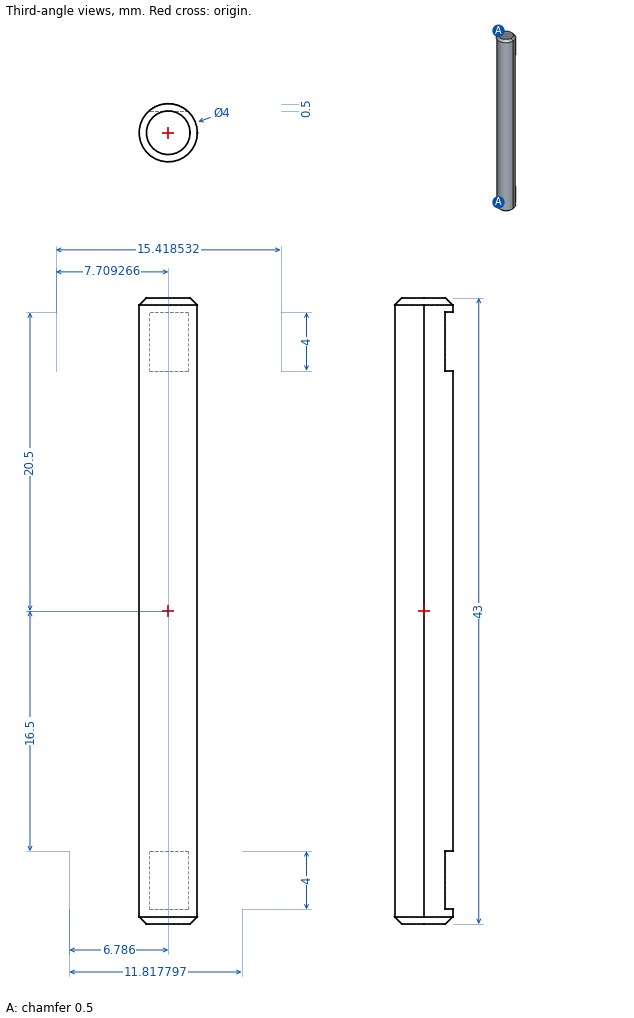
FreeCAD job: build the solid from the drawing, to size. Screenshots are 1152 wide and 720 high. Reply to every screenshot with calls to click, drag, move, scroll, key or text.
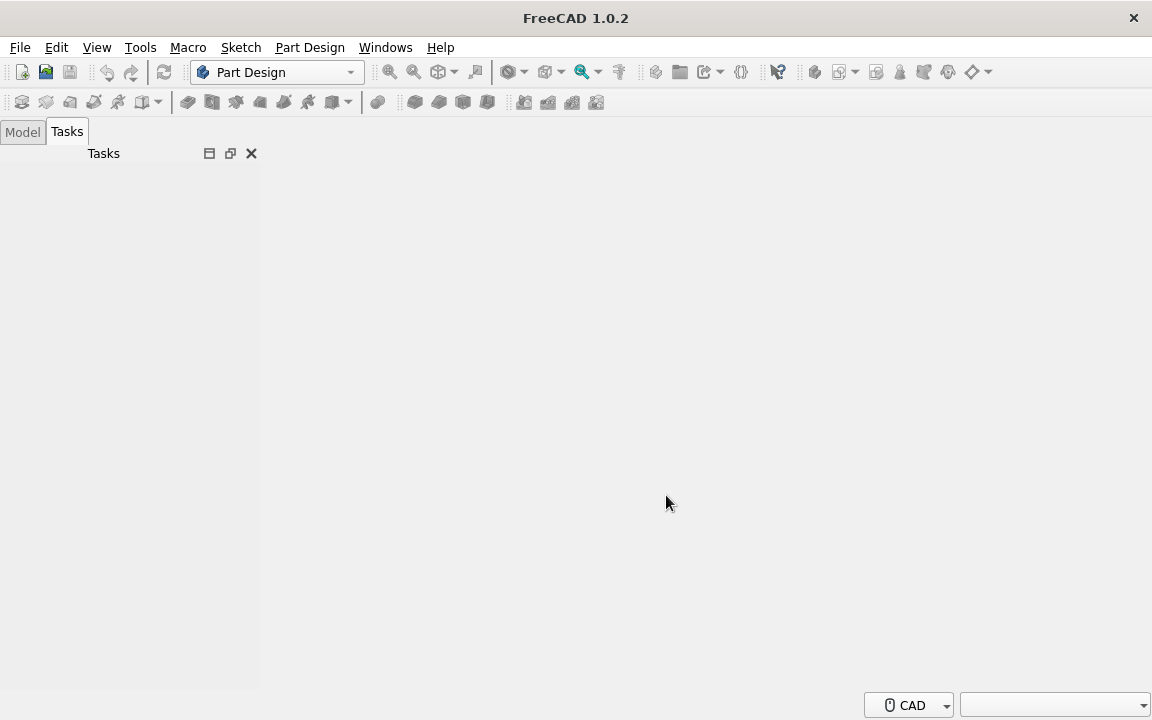
key(ctrl+n)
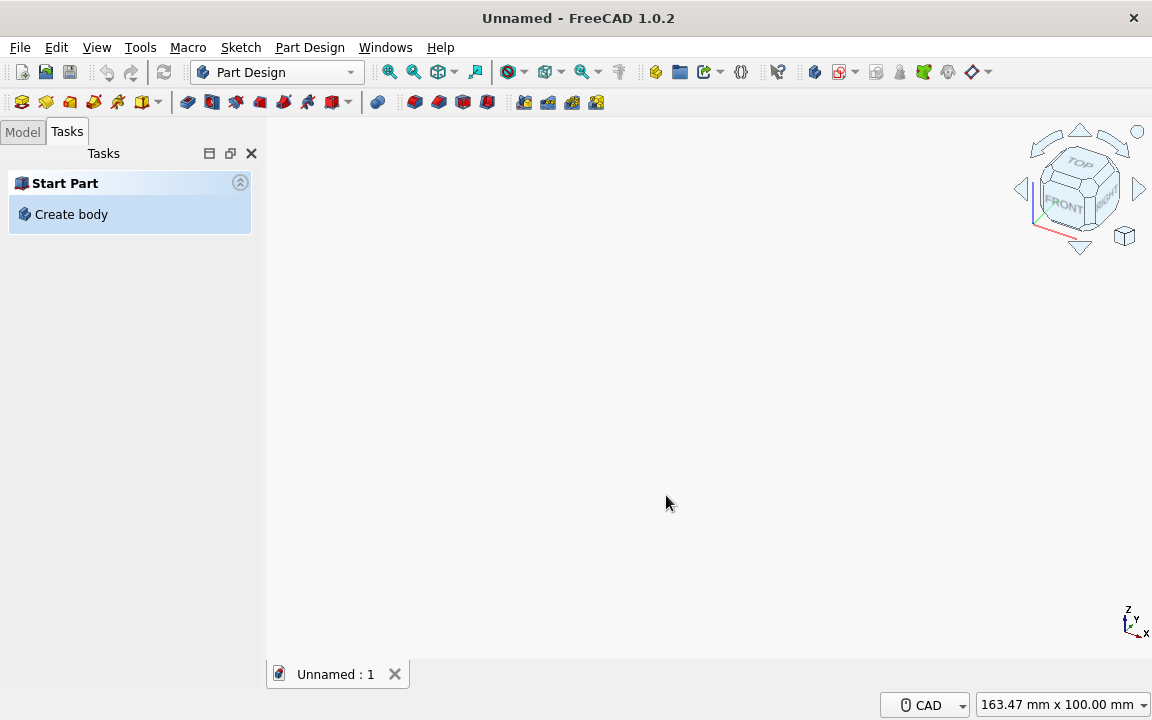
click(840, 72)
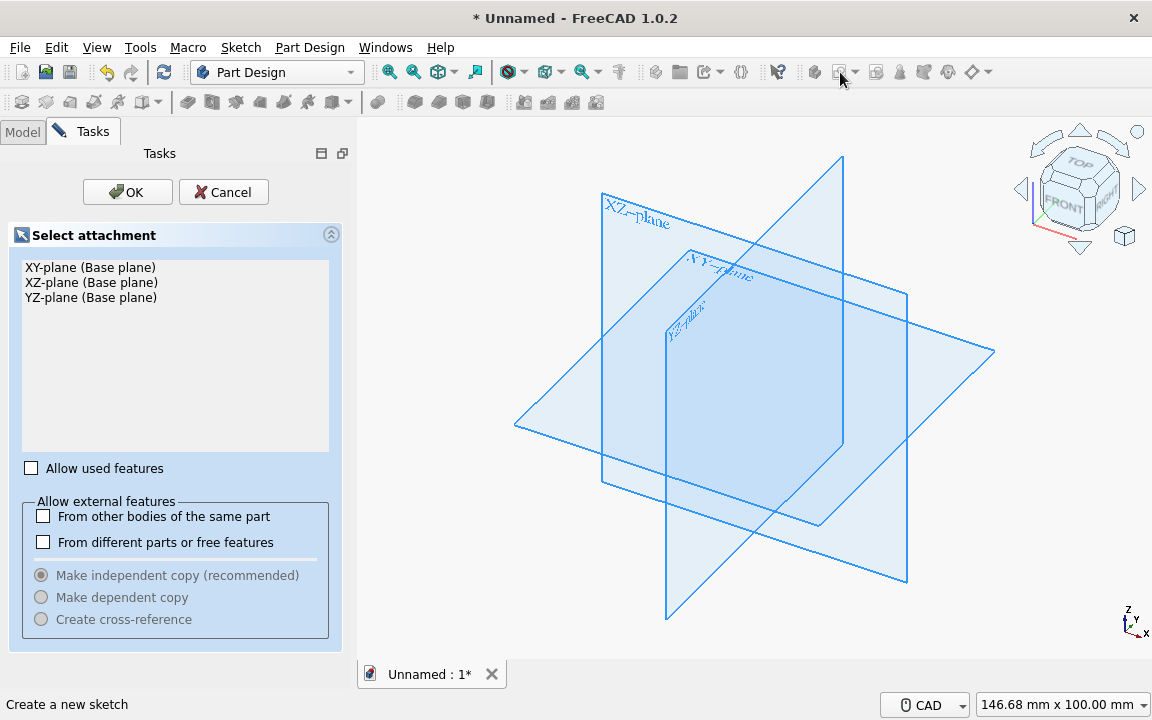
click(82, 268)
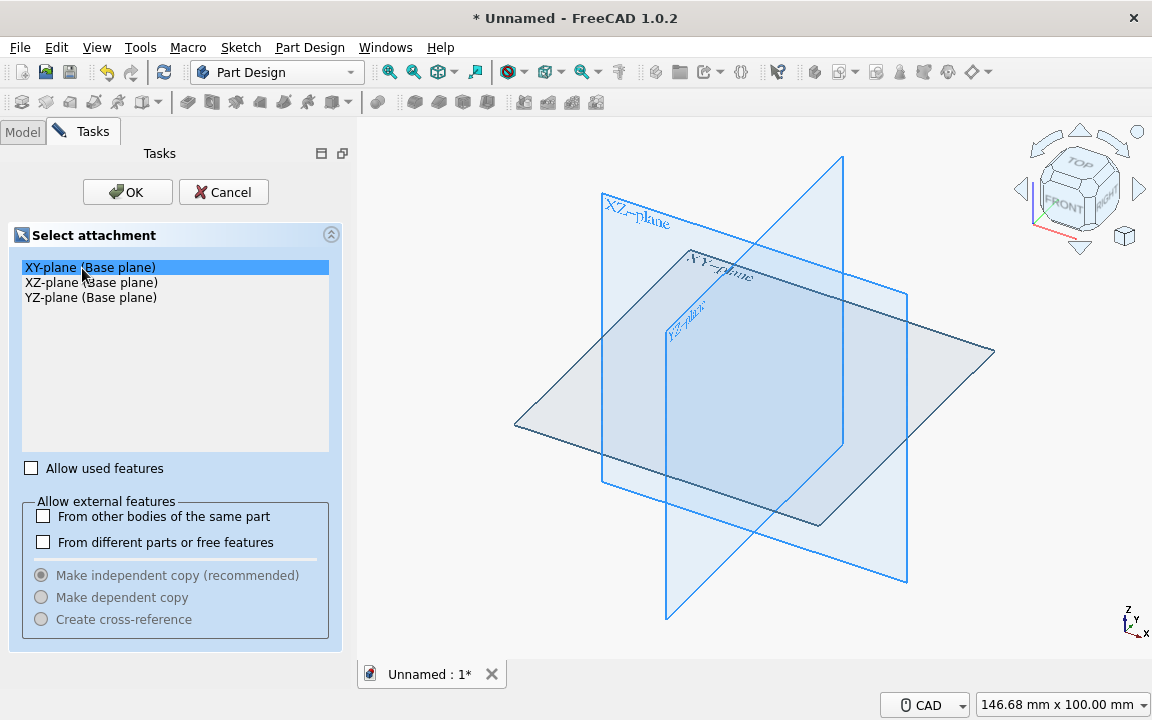
click(128, 192)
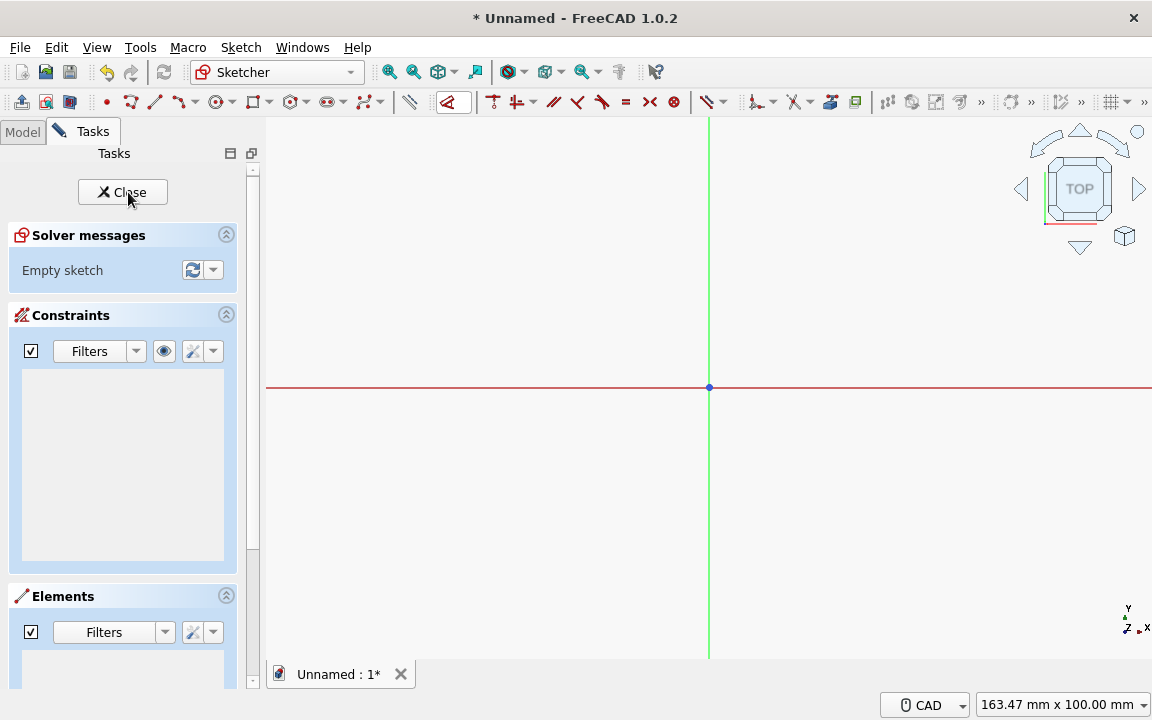
scroll(713, 388, up, 14)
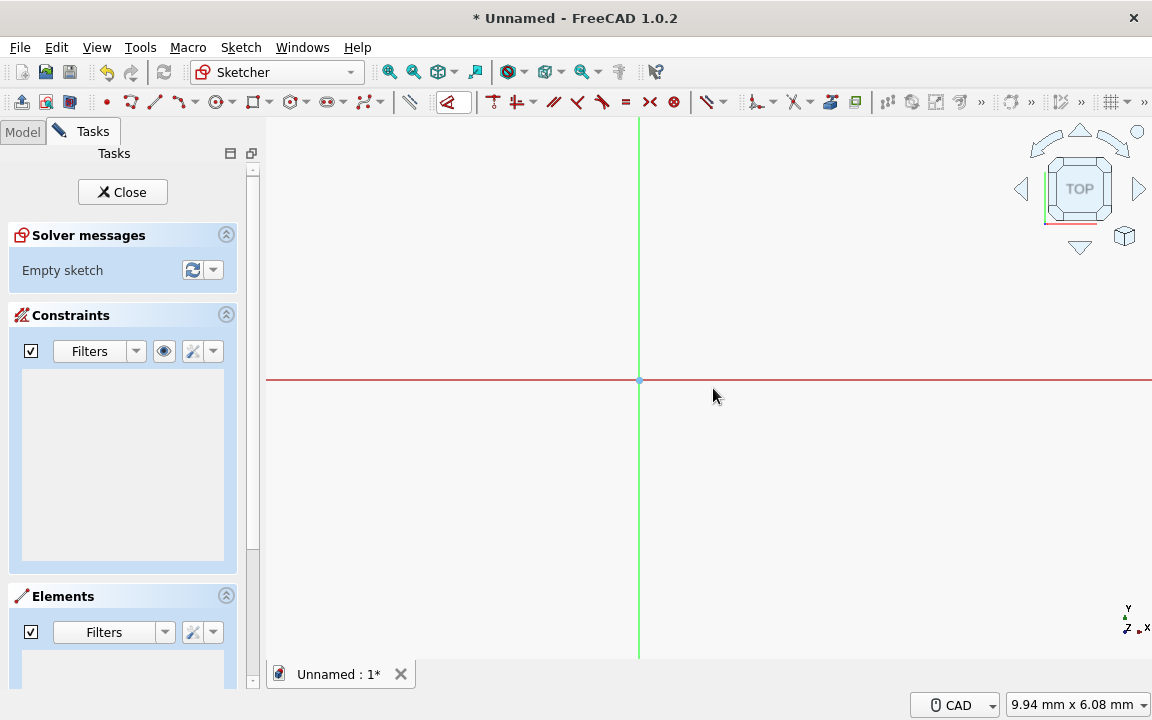
key(g)
key(c)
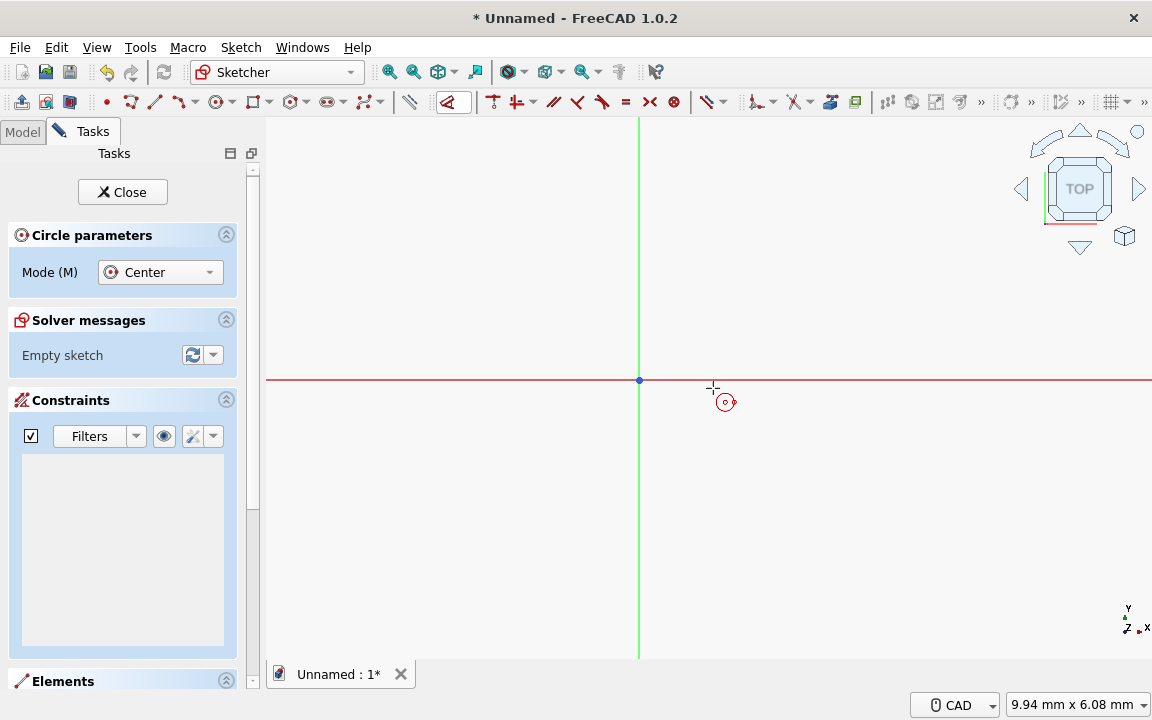
click(639, 380)
move(765, 254)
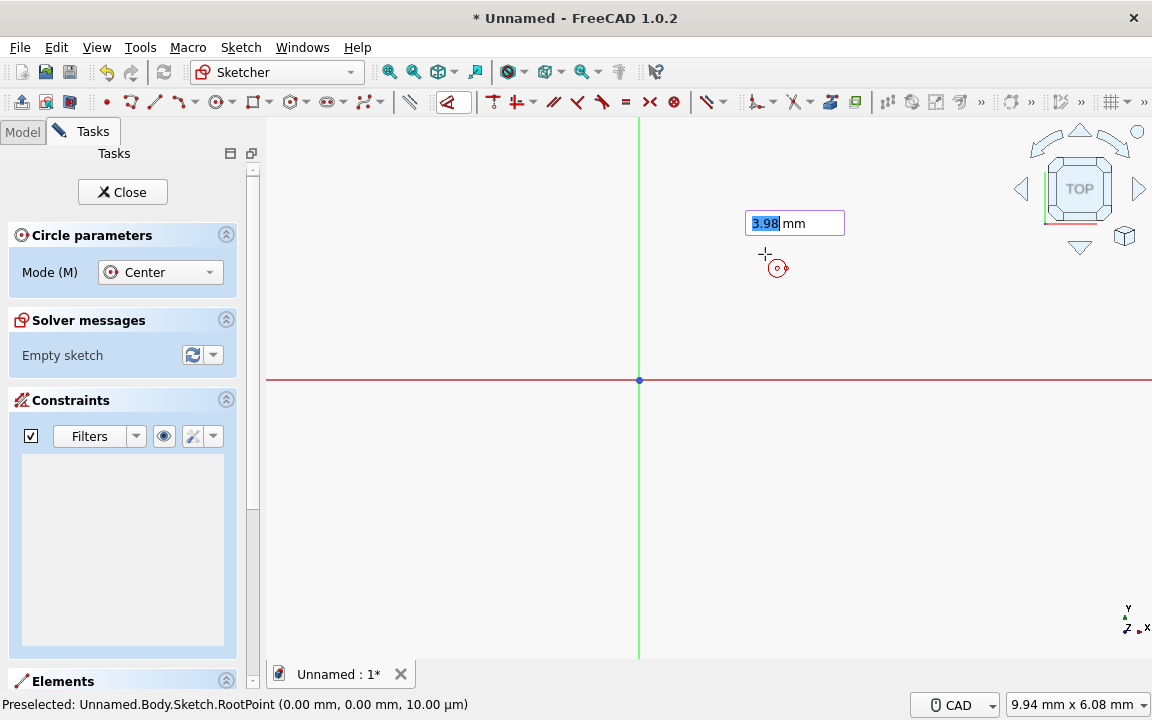
text(4)
key(Return)
key(Escape)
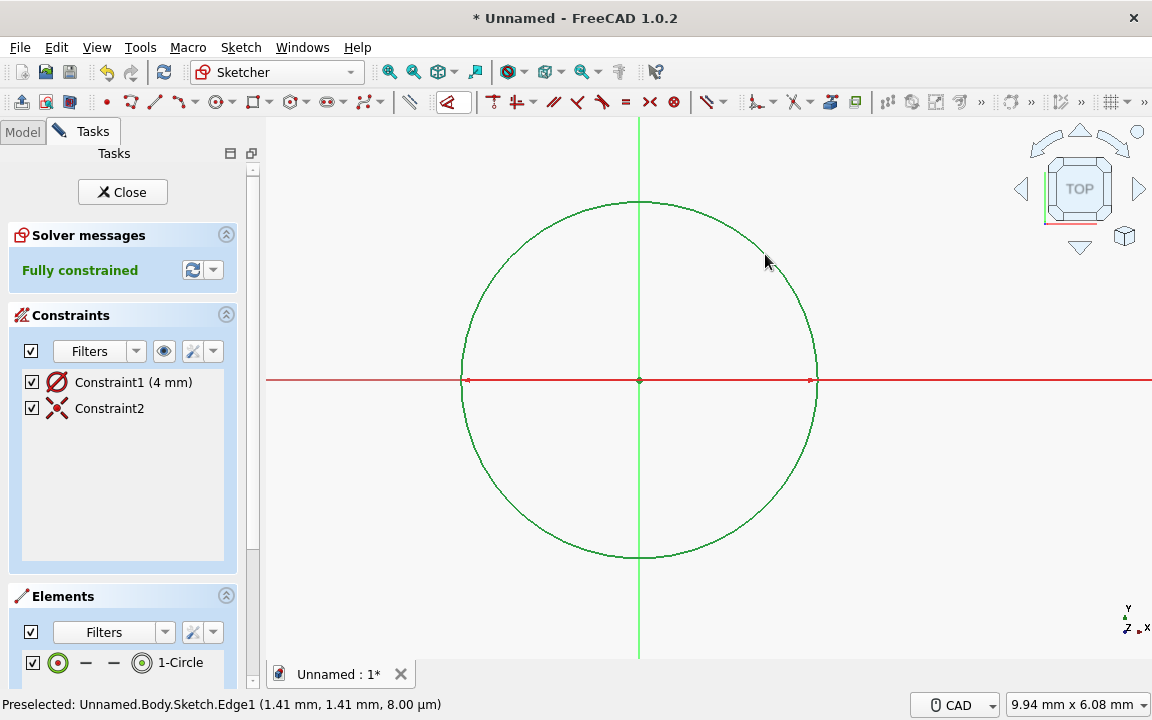
click(123, 192)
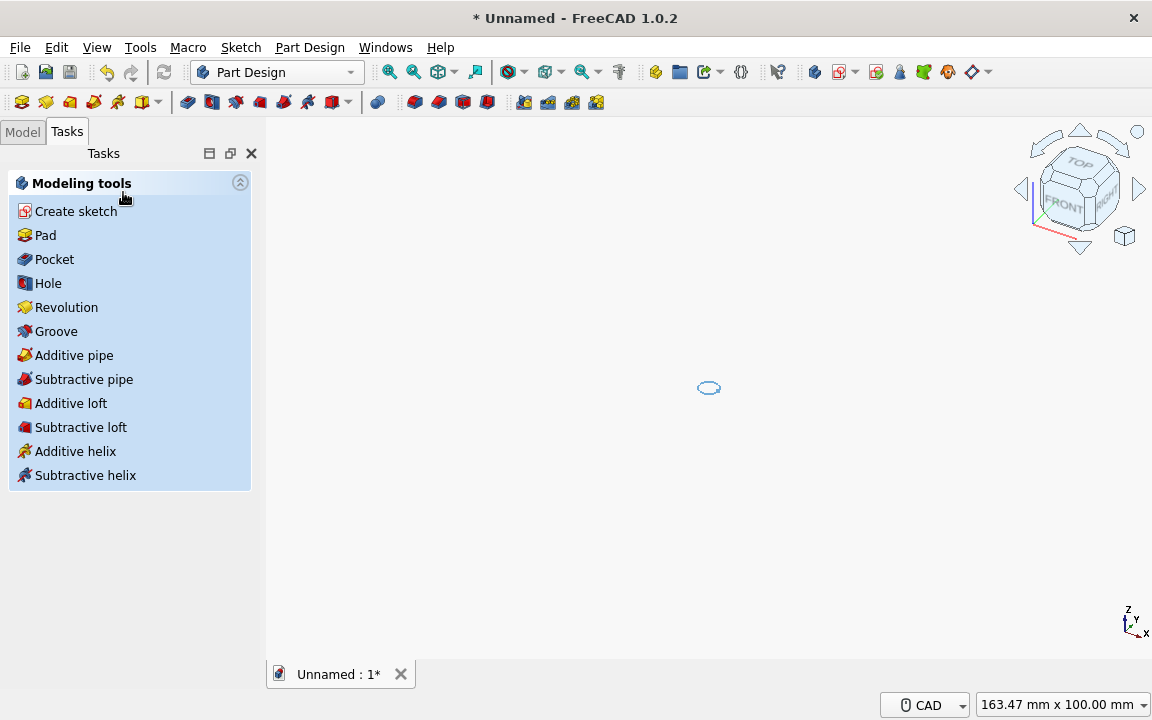
click(22, 102)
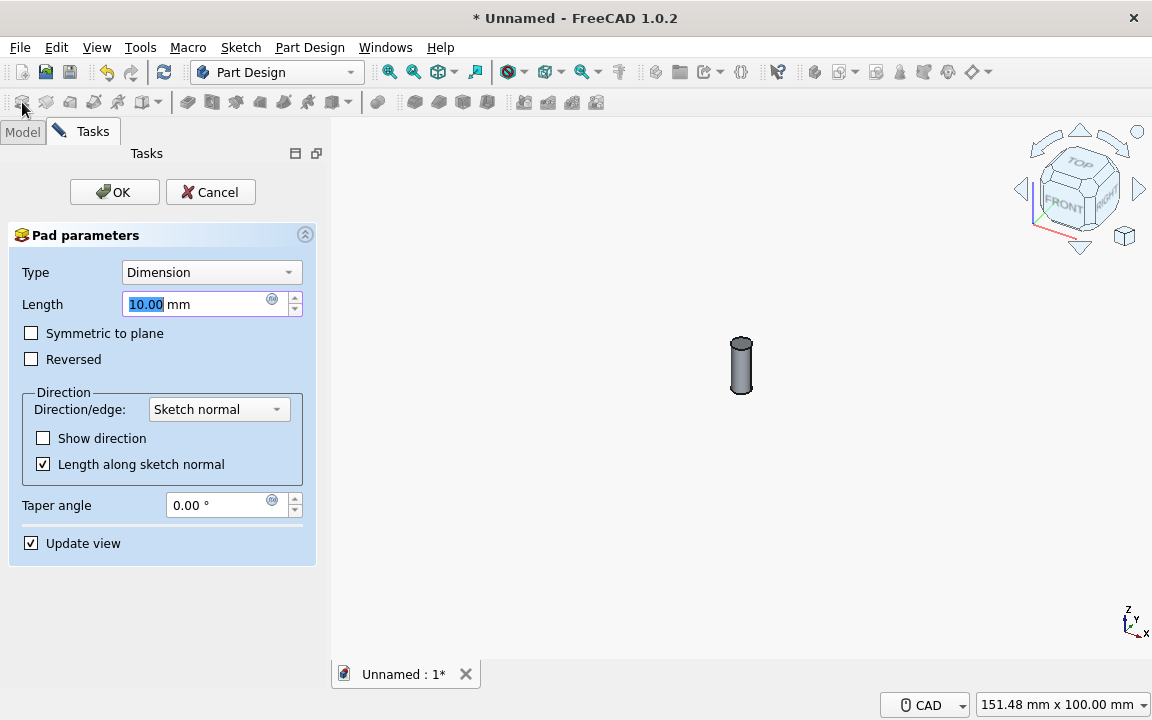
text(43)
key(Tab)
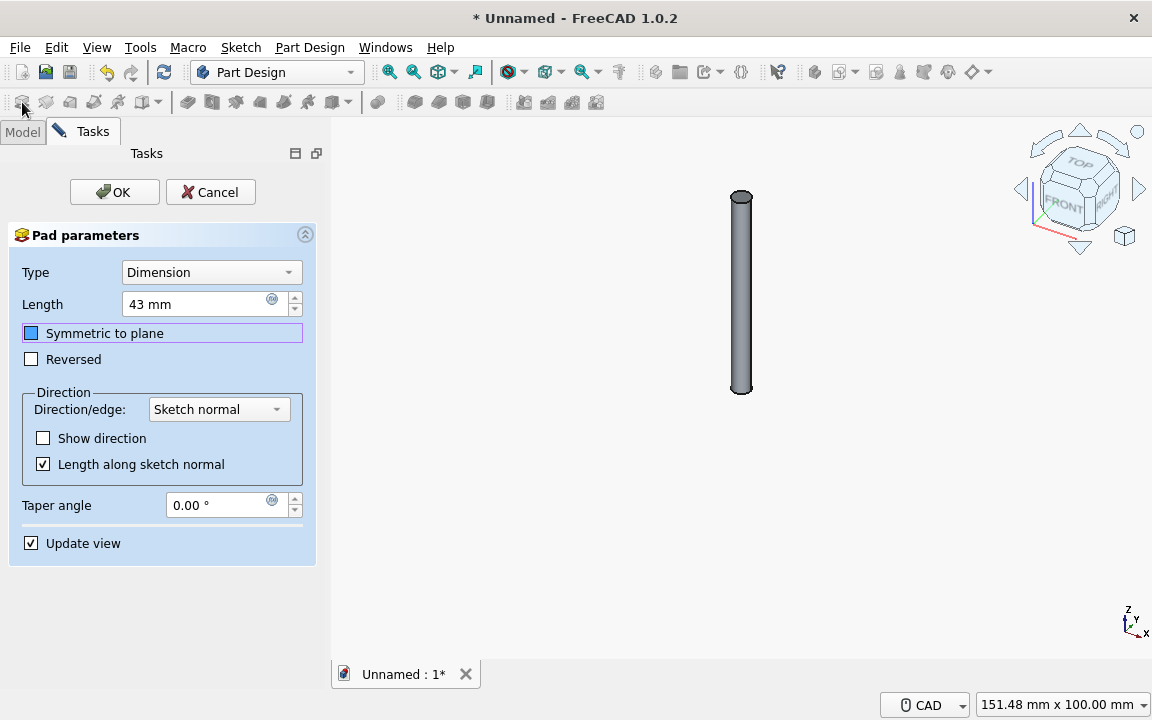
click(30, 333)